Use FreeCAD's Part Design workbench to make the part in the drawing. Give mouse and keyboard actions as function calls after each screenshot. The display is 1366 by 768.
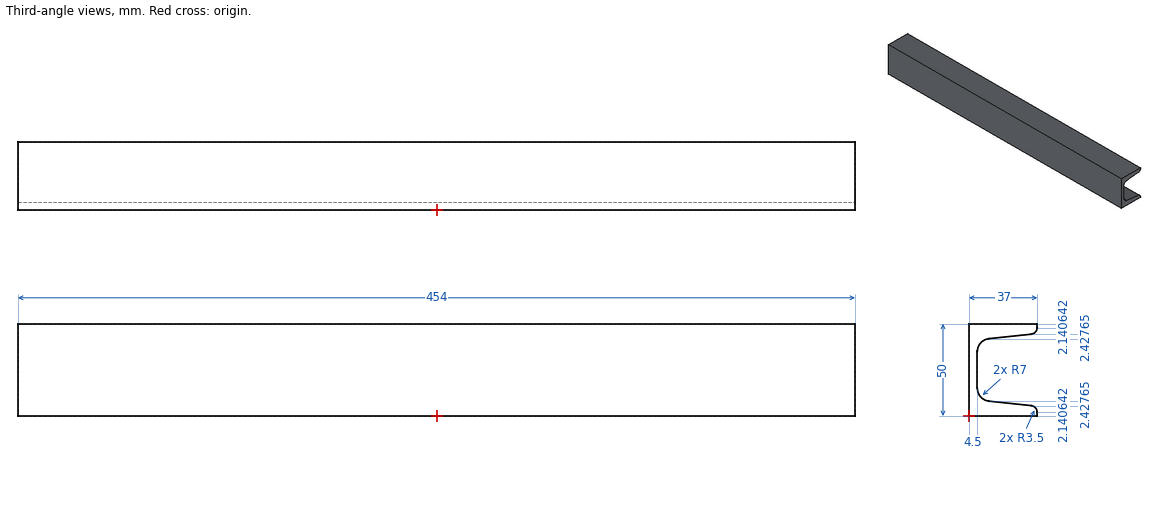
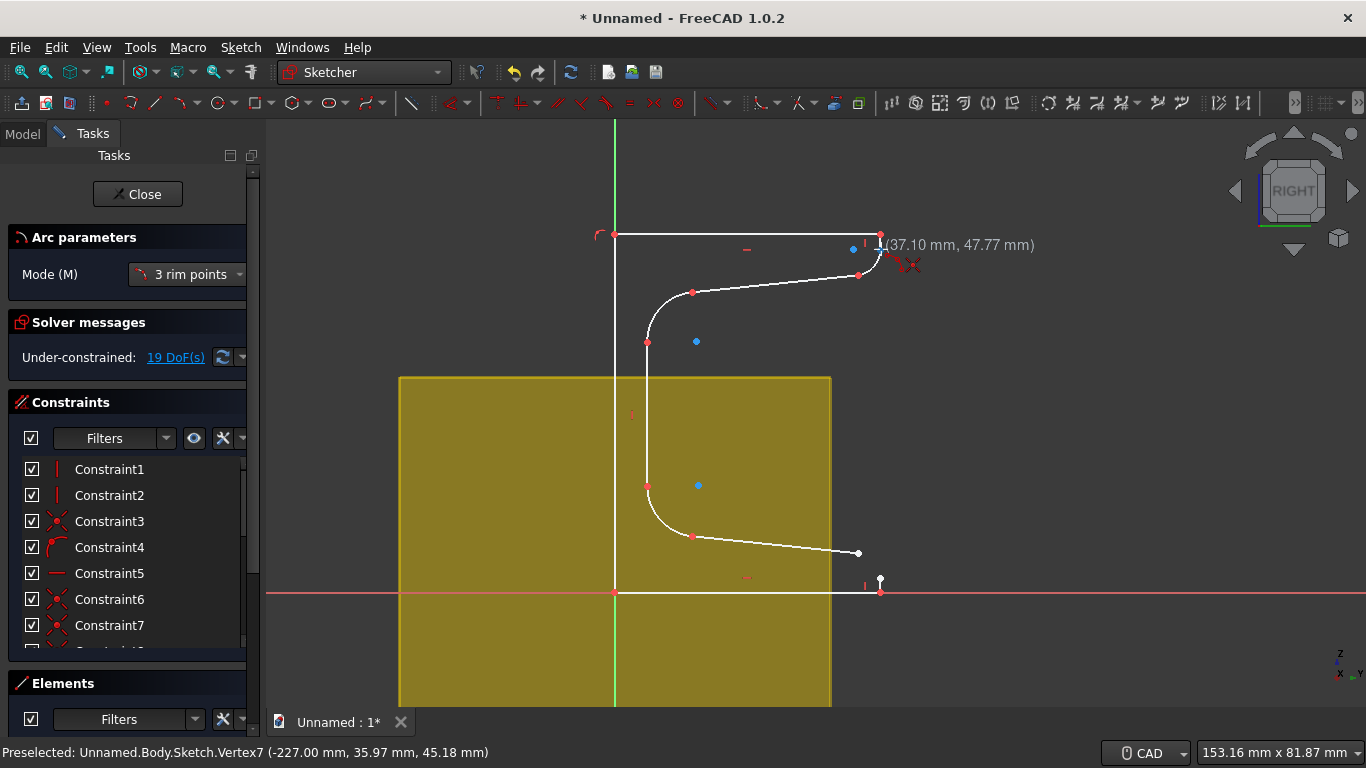
scroll(881, 577, up, 4)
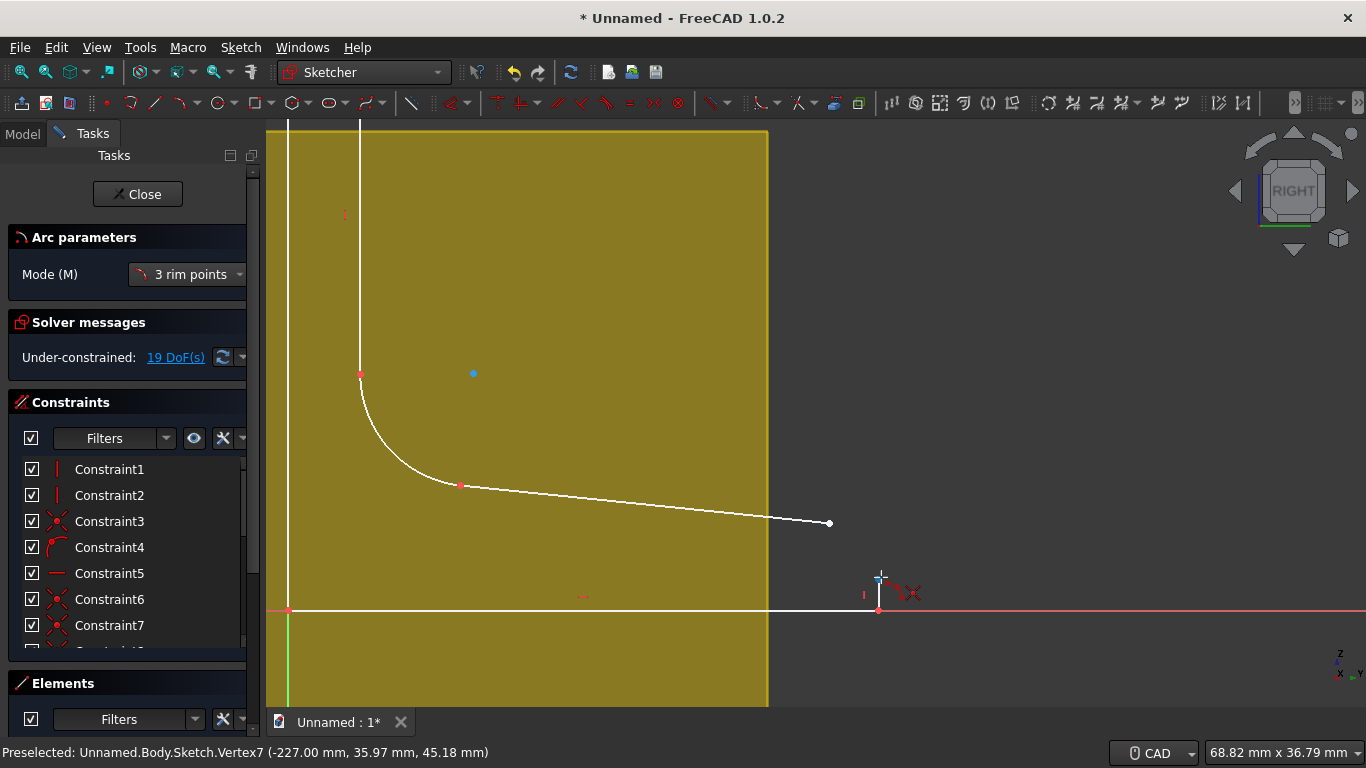
click(879, 579)
click(830, 523)
click(865, 539)
key(Escape)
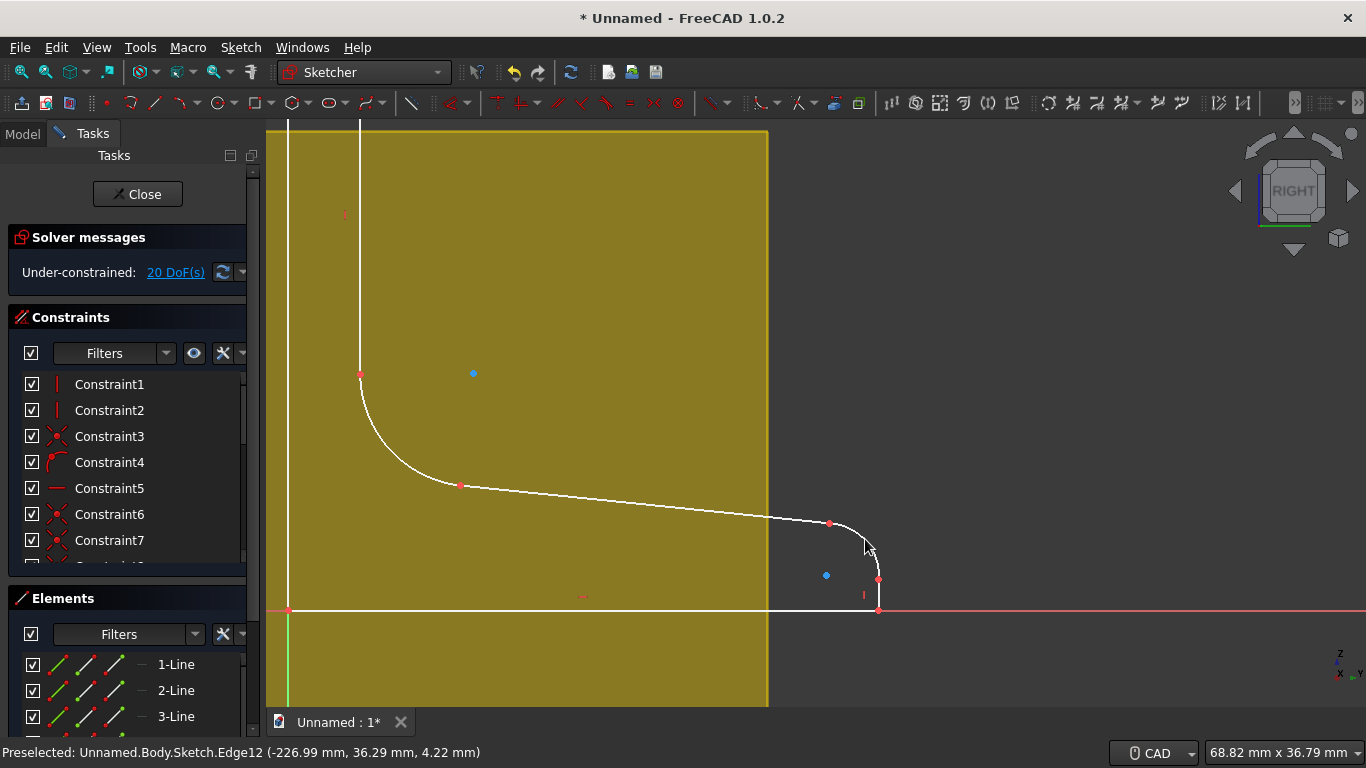
click(719, 512)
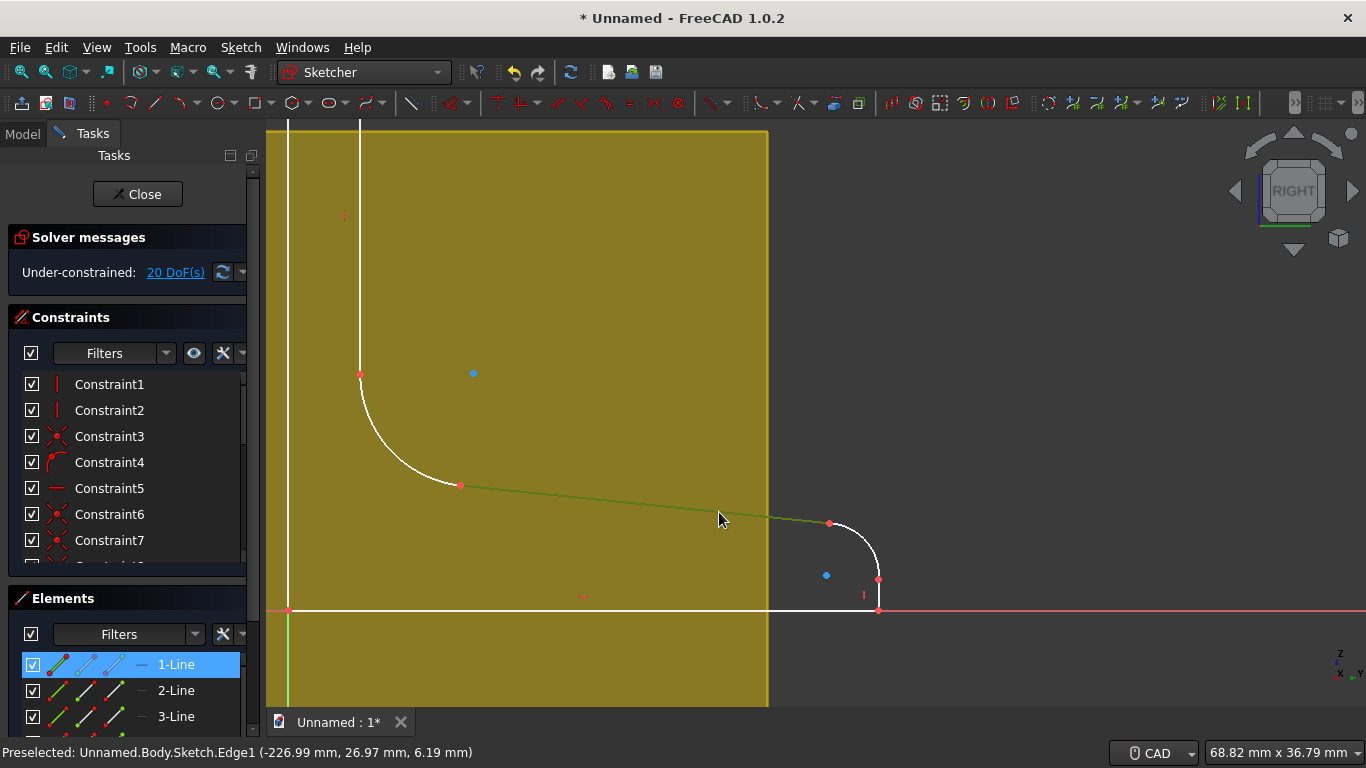
click(371, 422)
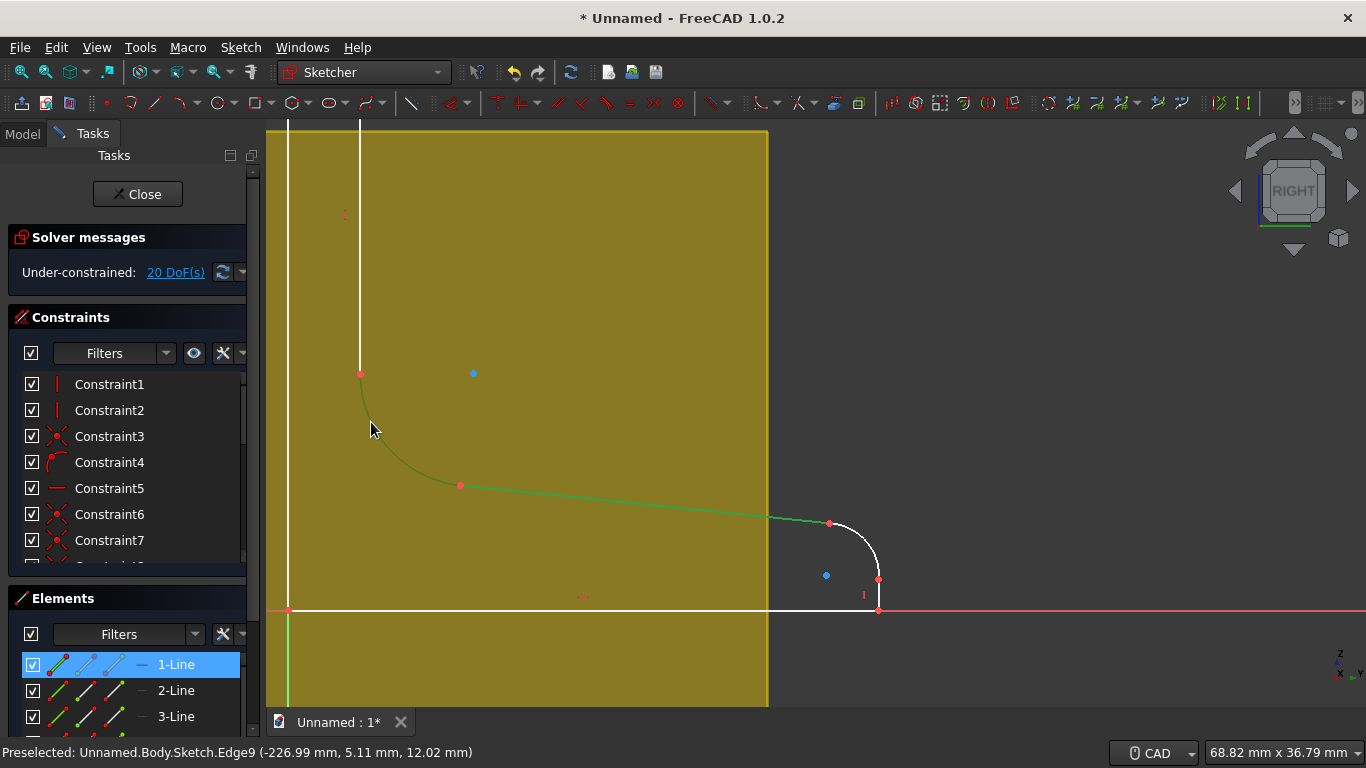
click(606, 104)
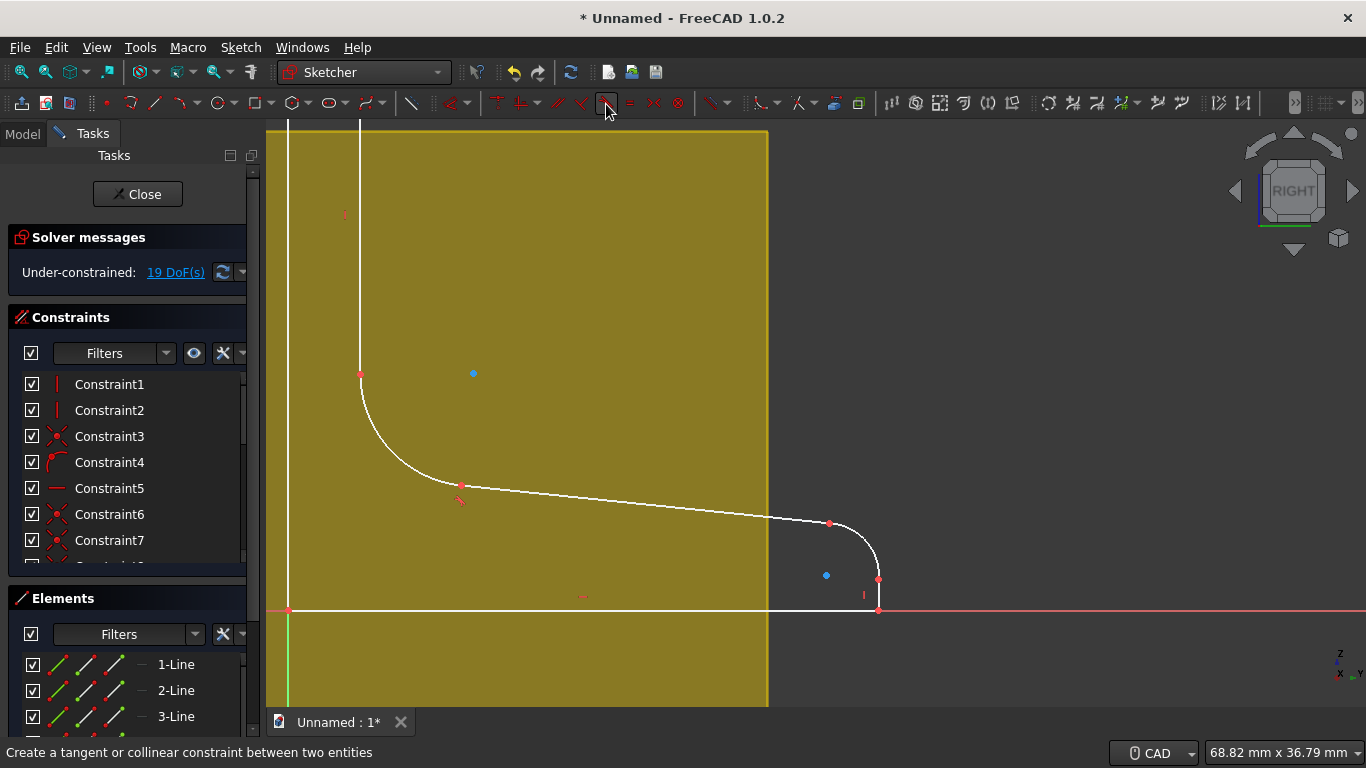
click(719, 512)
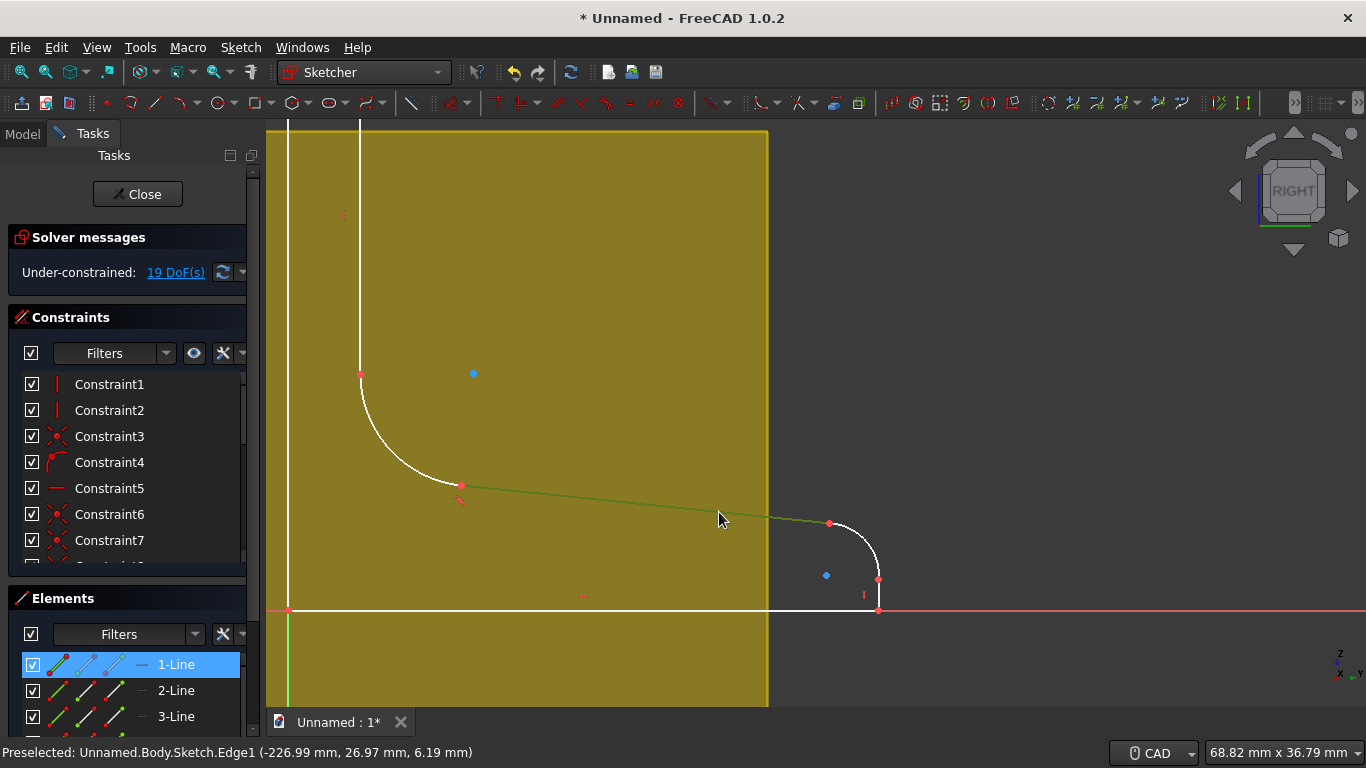
click(875, 555)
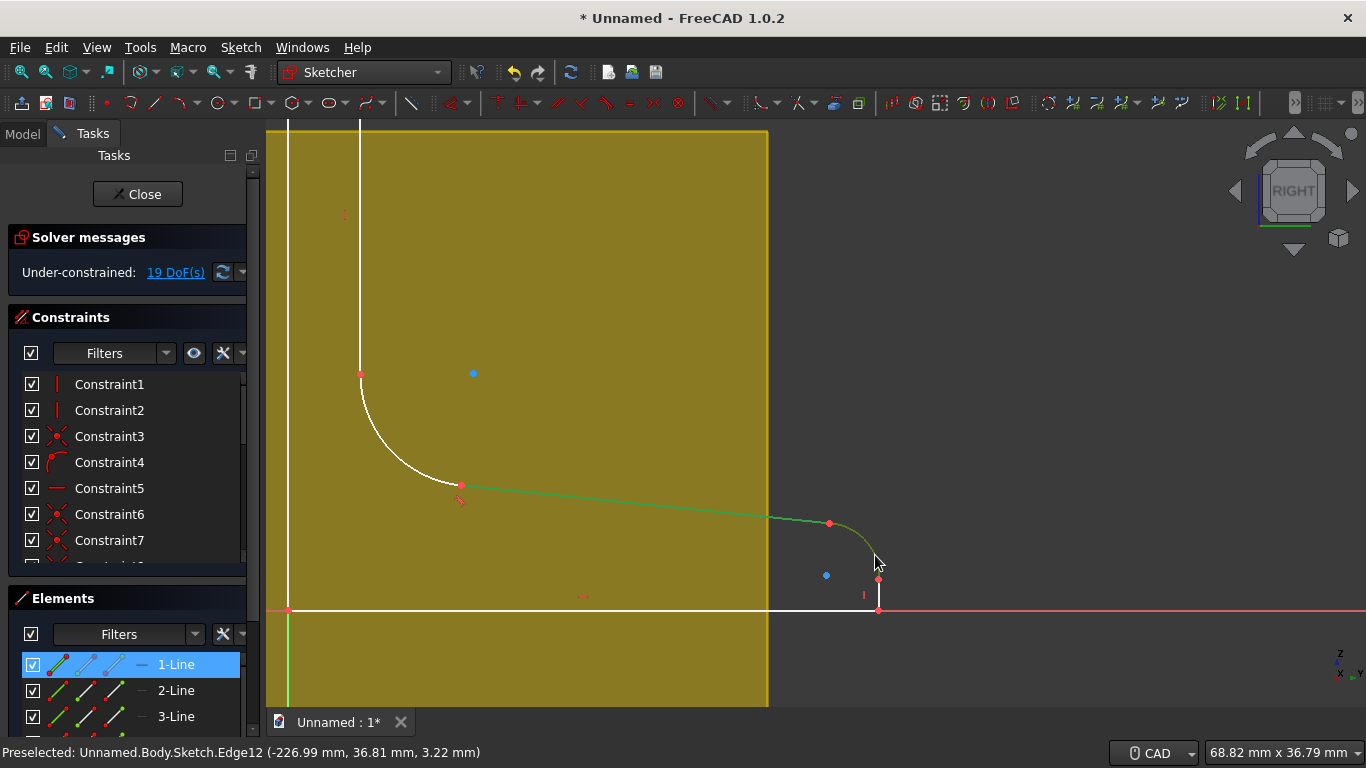
key(t)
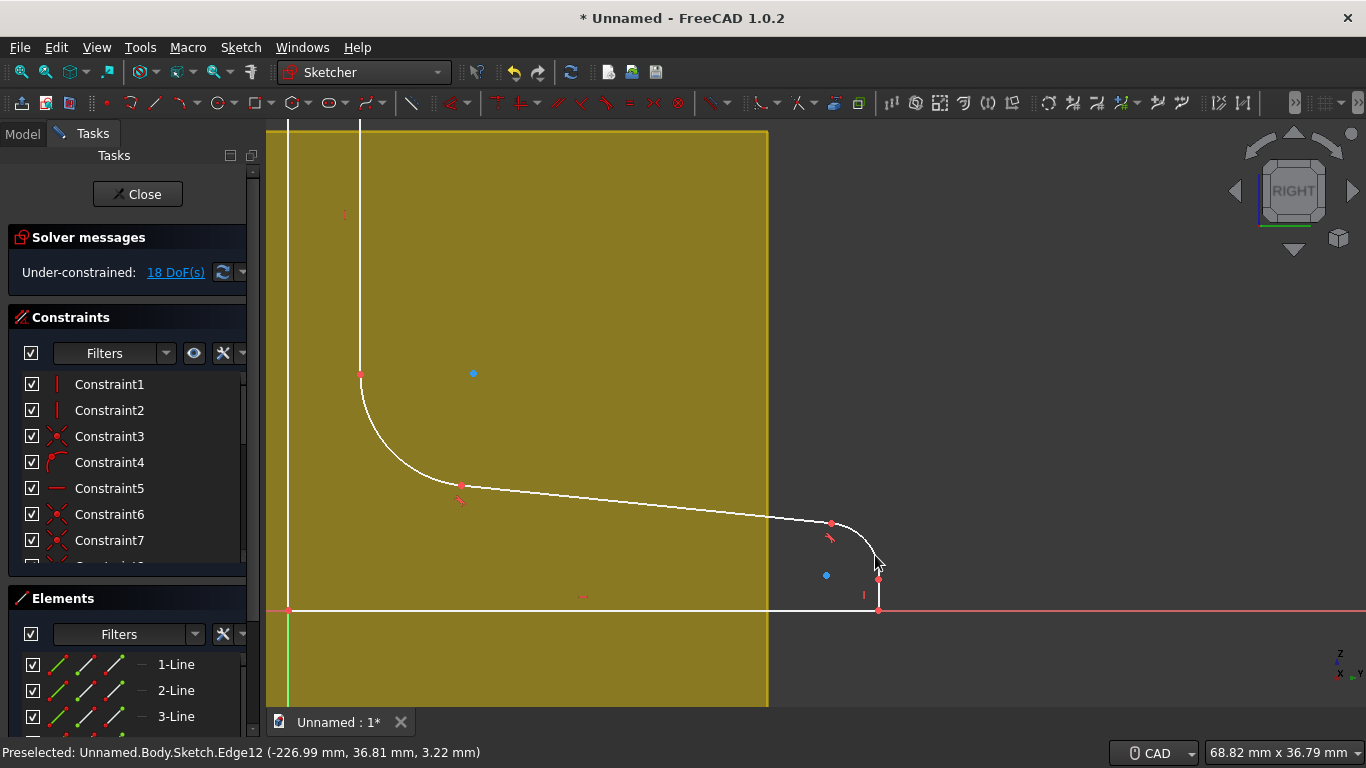
click(360, 278)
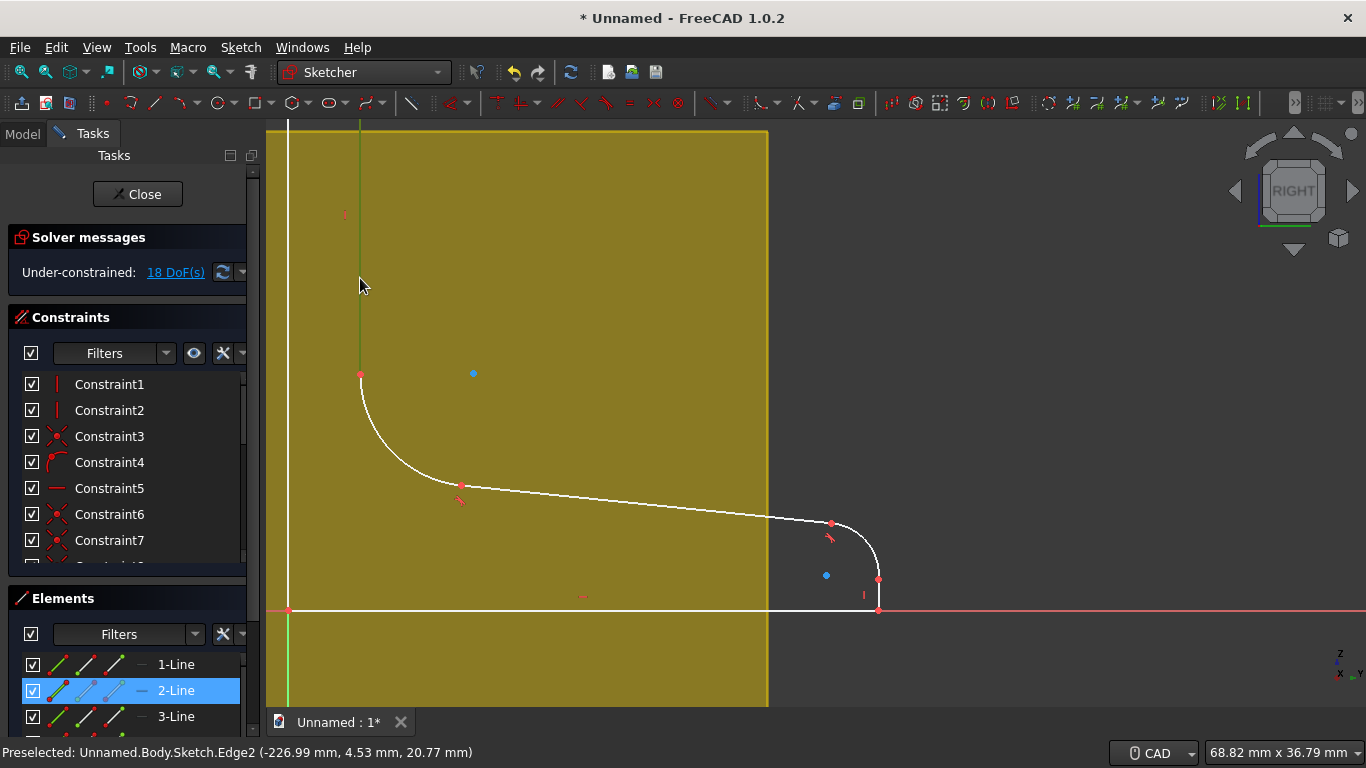
click(371, 422)